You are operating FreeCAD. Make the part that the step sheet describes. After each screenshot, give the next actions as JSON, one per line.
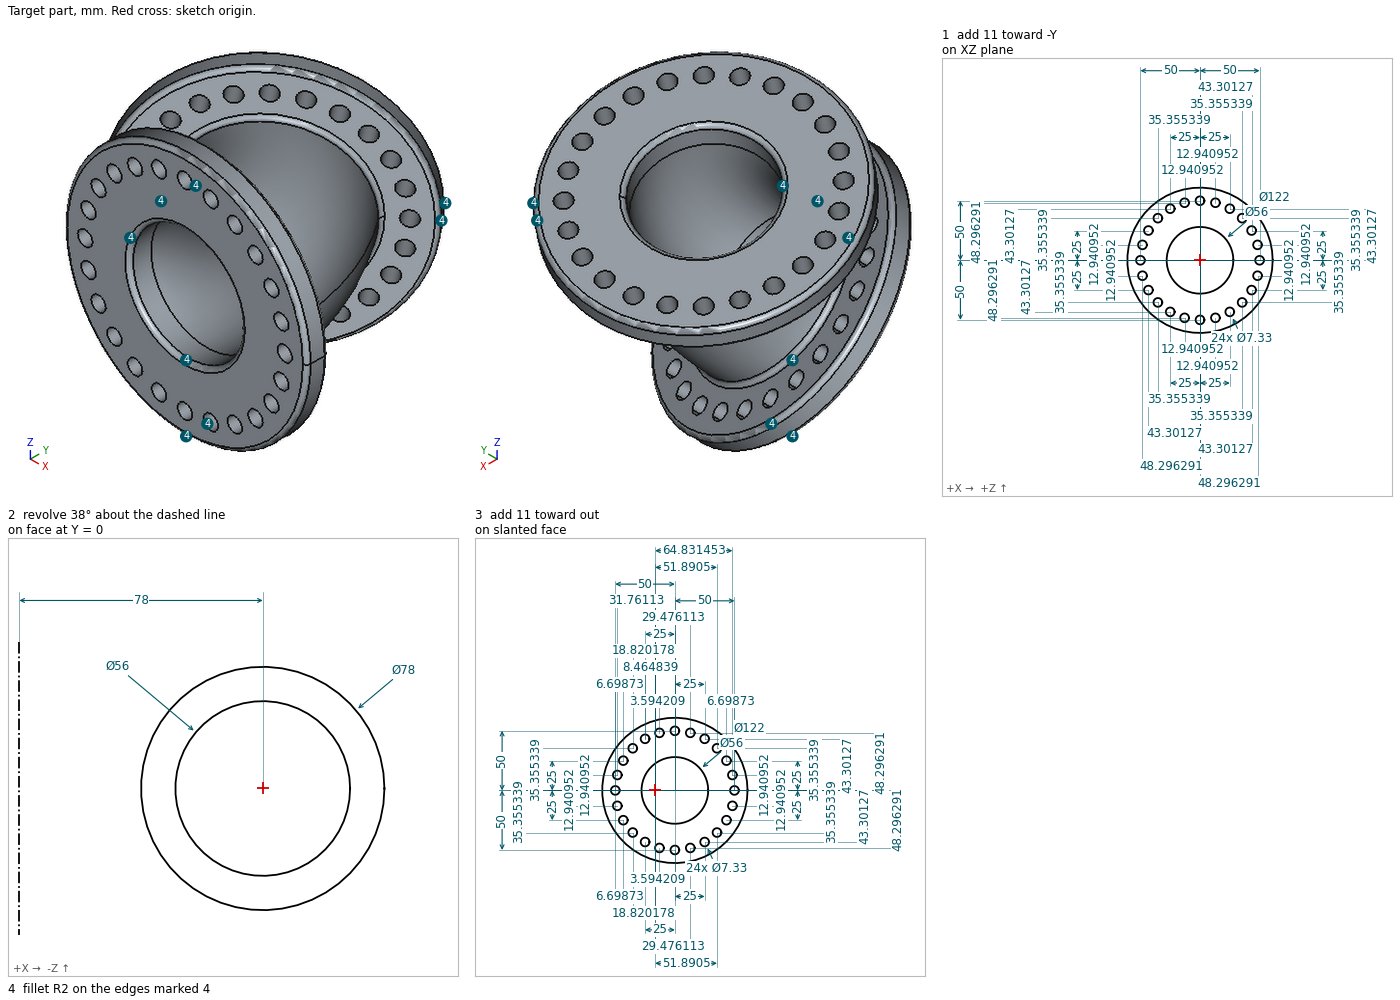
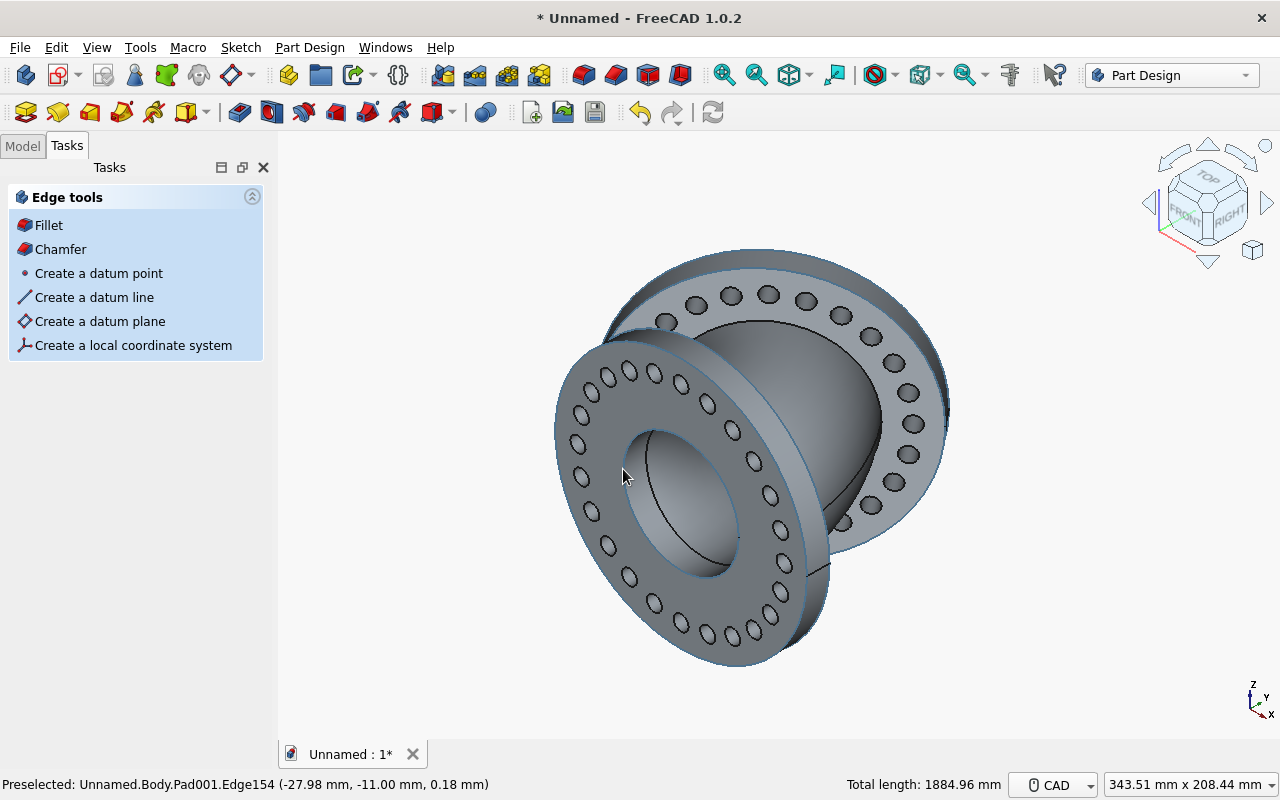
{"action": "key", "text": "2"}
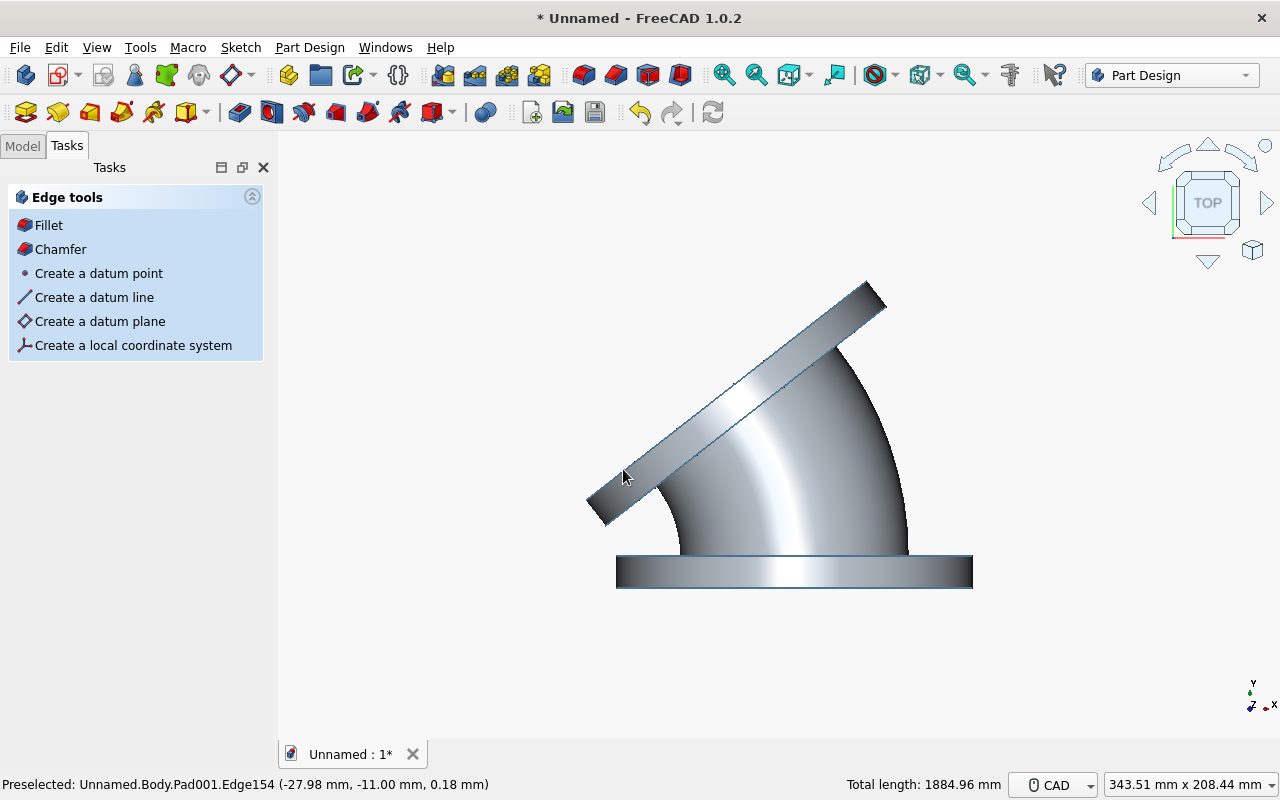
{"action": "key", "text": "1"}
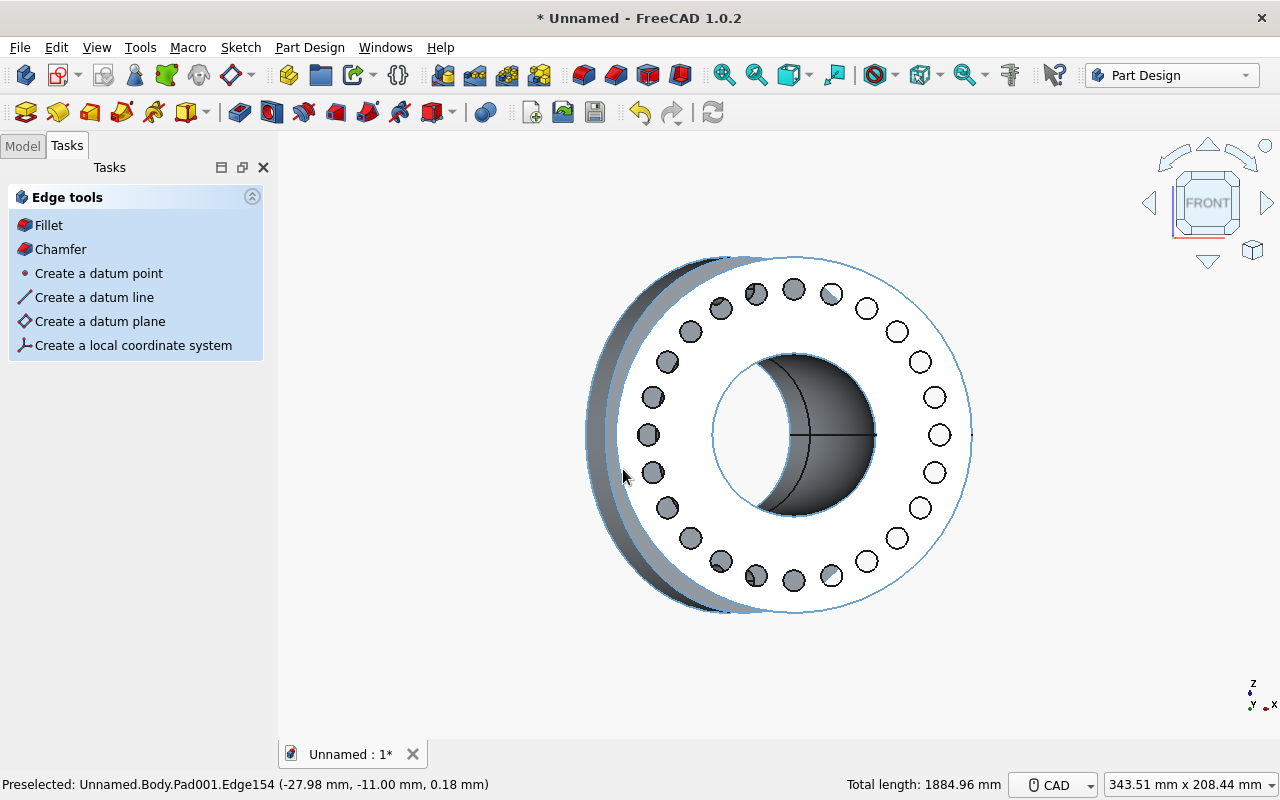
{"action": "key", "text": "3"}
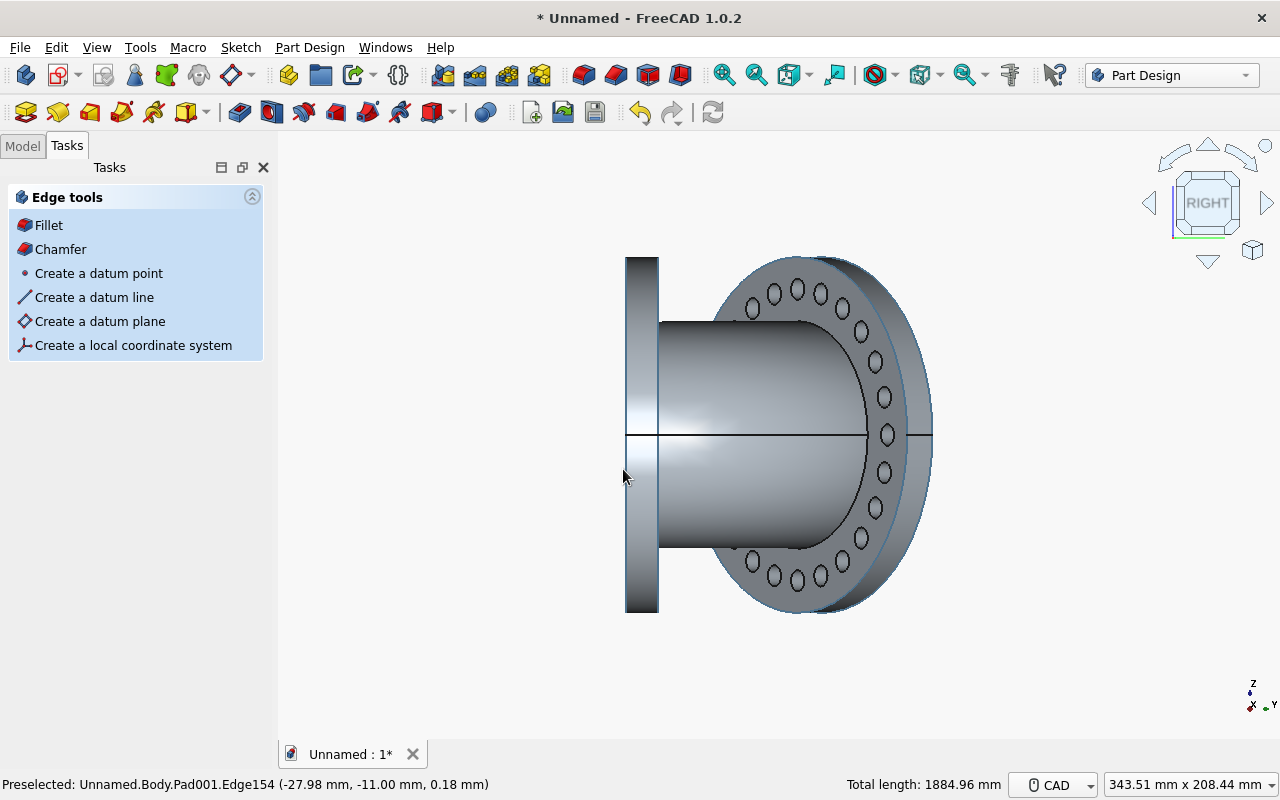
{"action": "key", "text": "5"}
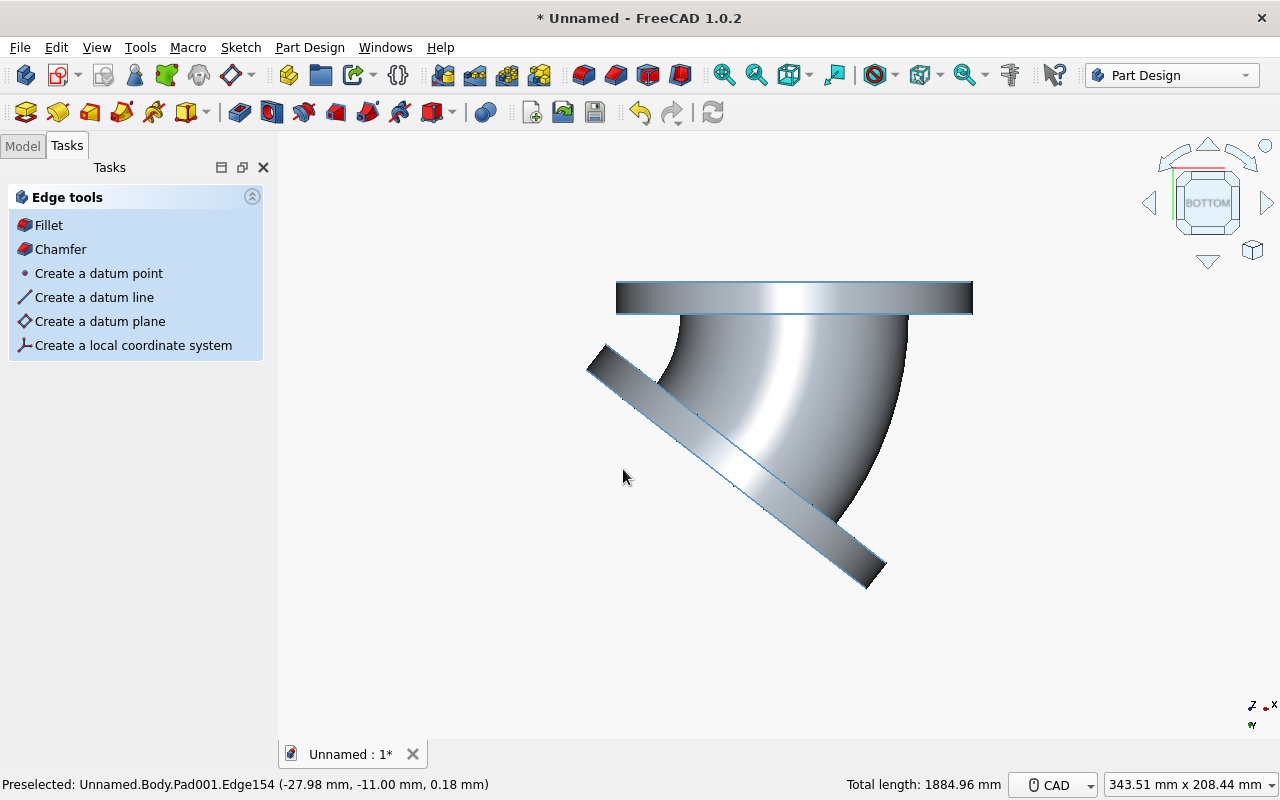
{"action": "key", "text": "4"}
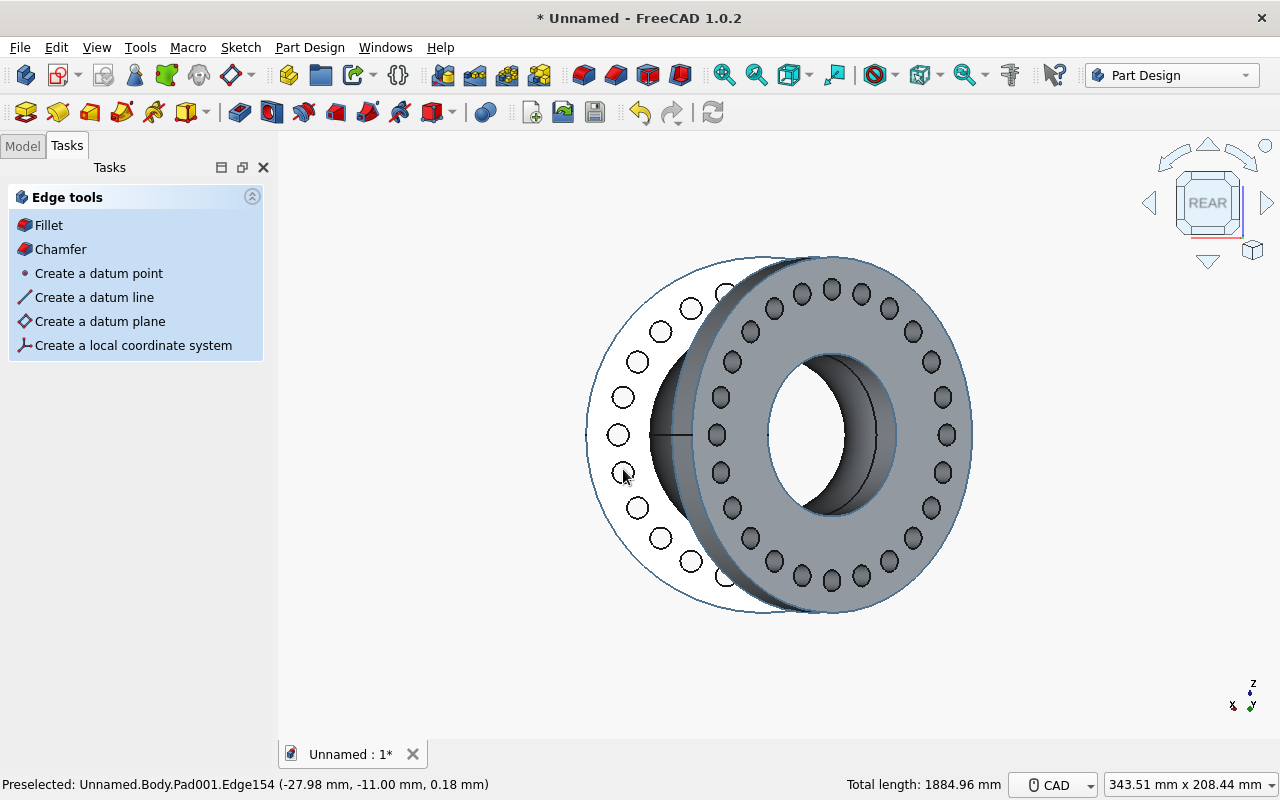
{"action": "key", "text": "6"}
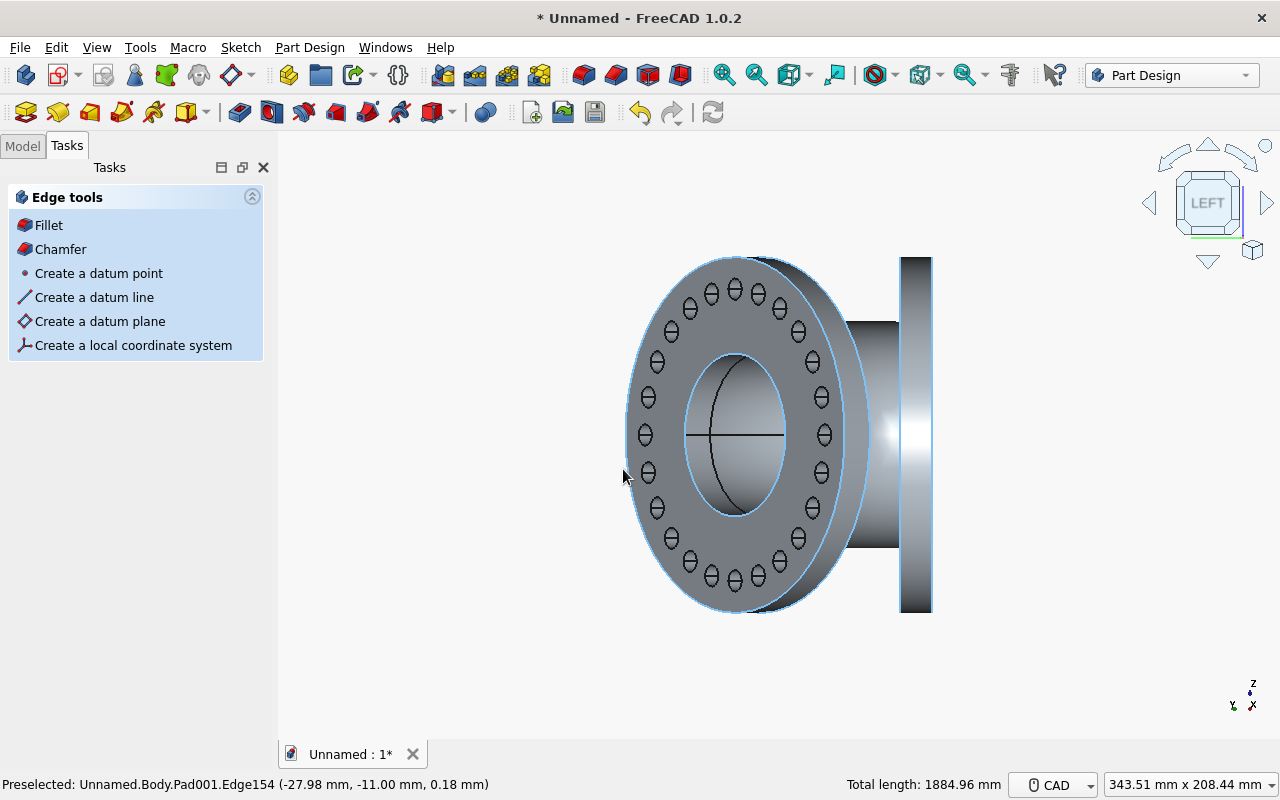
{"action": "key", "text": "v 3"}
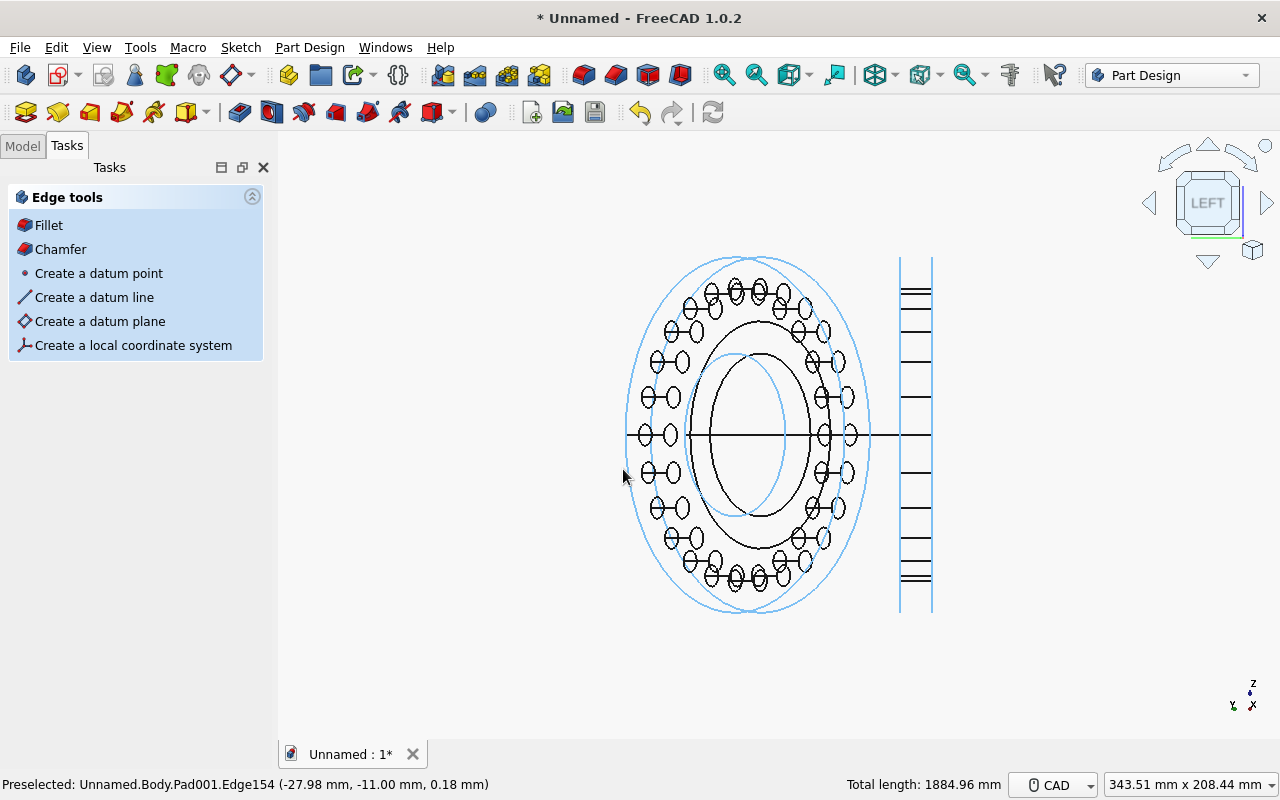
{"action": "key", "text": "0"}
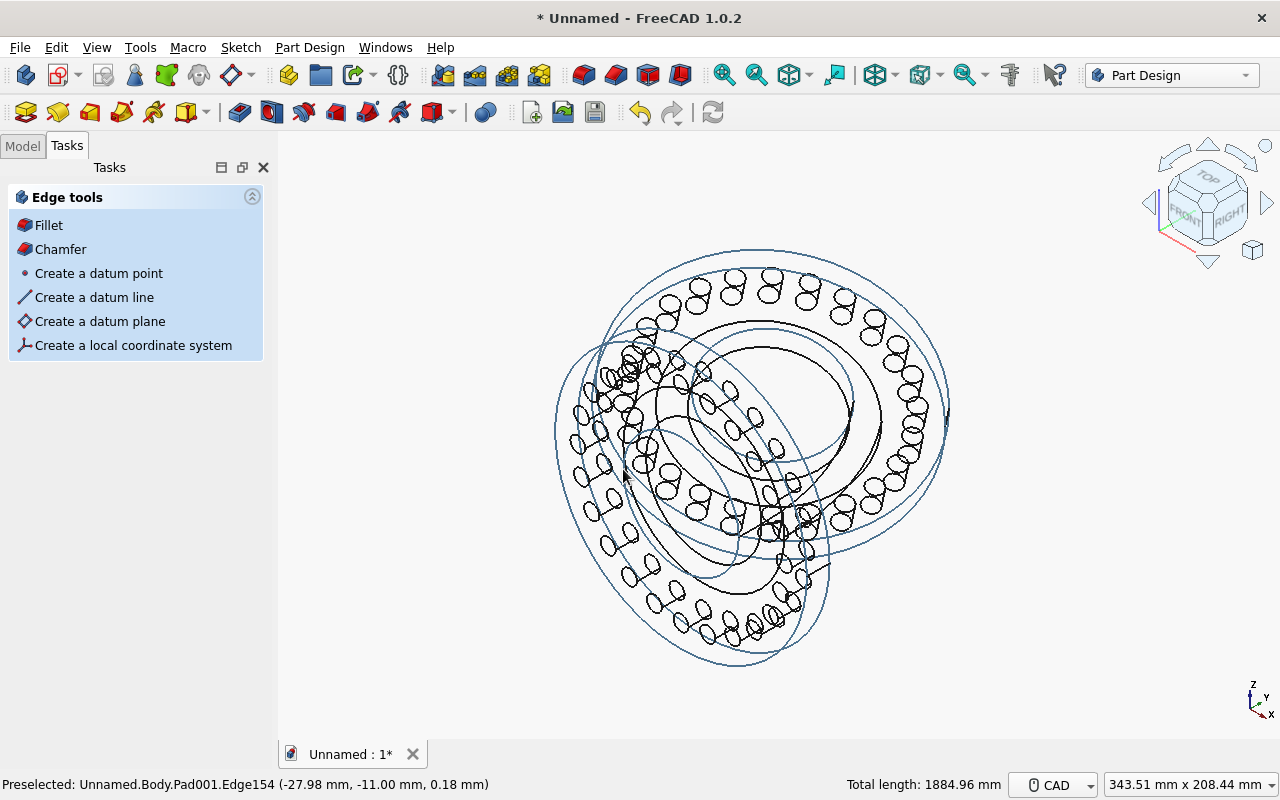
{"action": "left_click", "coordinate": [639, 507], "text": "ctrl"}